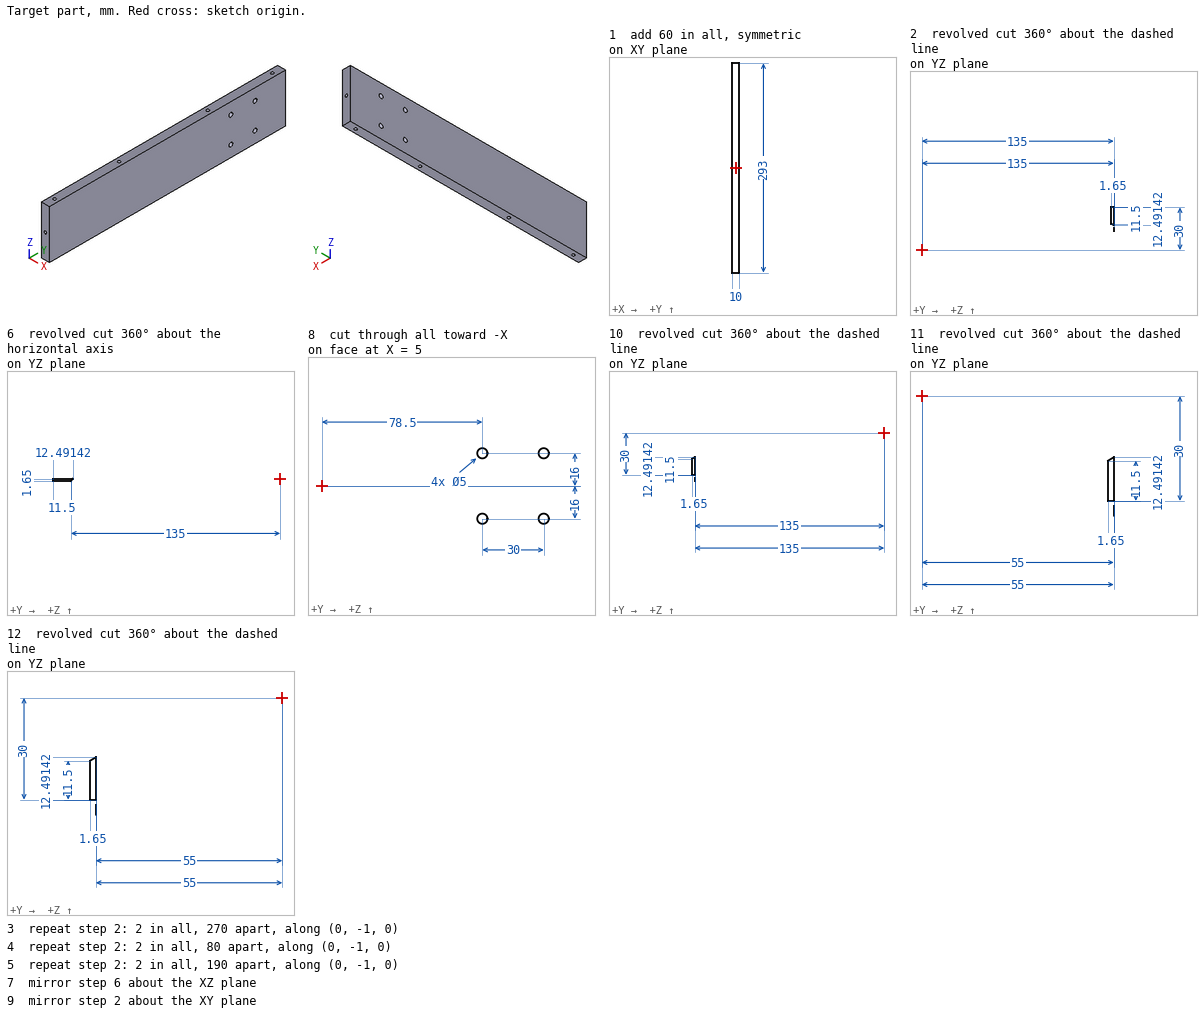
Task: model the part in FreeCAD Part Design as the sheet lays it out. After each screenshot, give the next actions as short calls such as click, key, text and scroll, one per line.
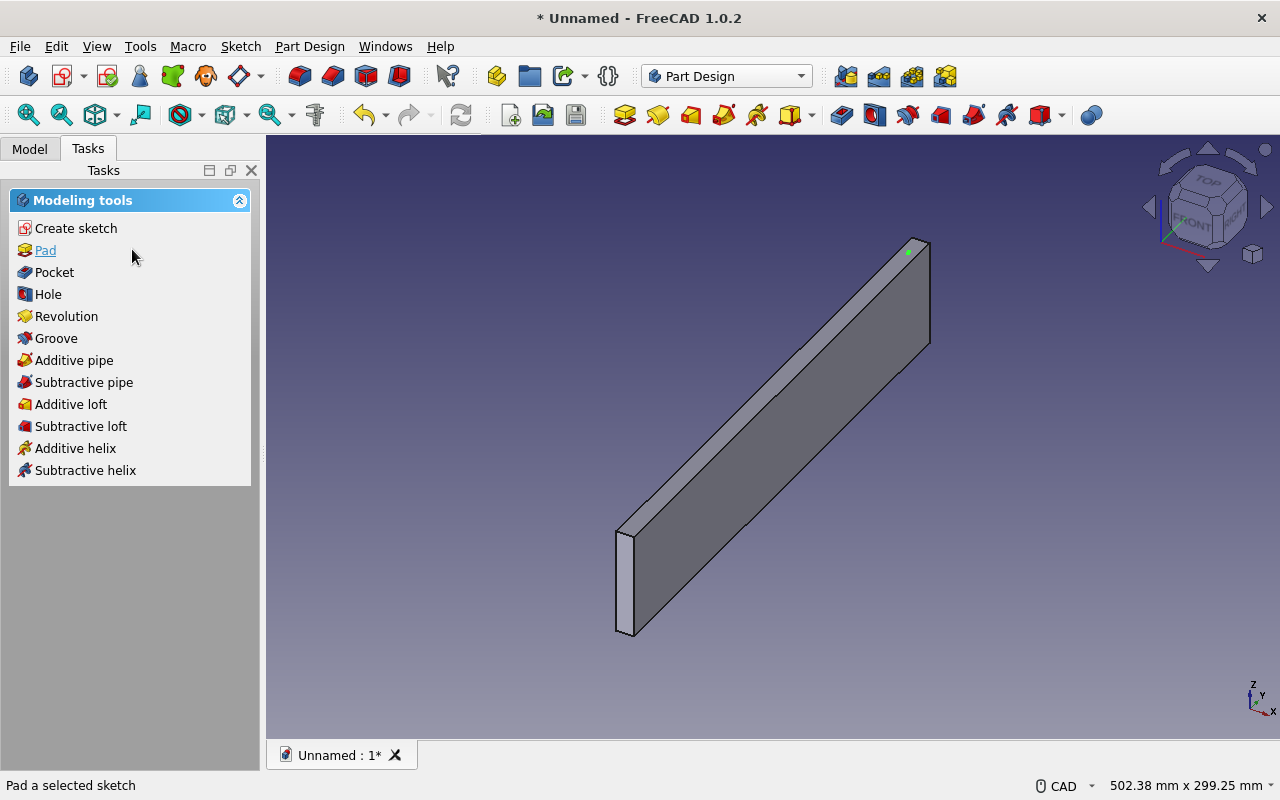
click(908, 116)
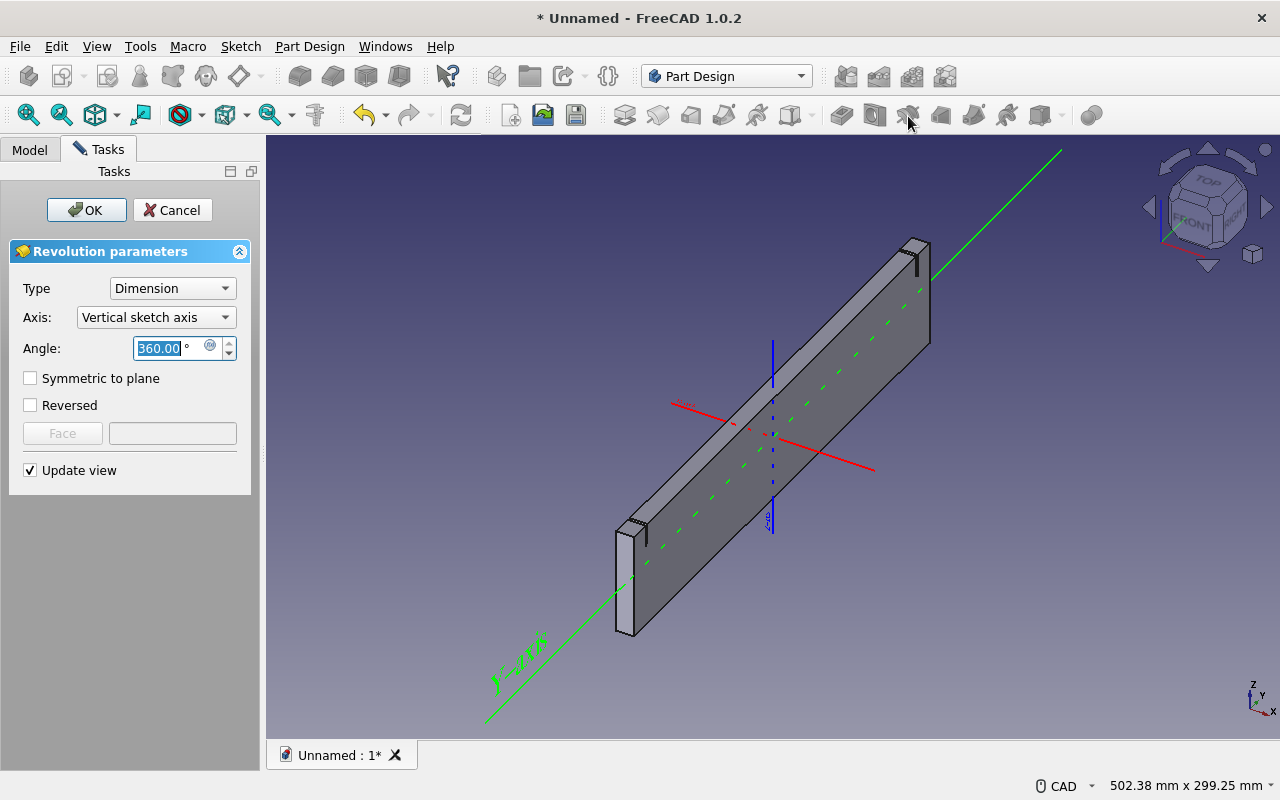
click(157, 318)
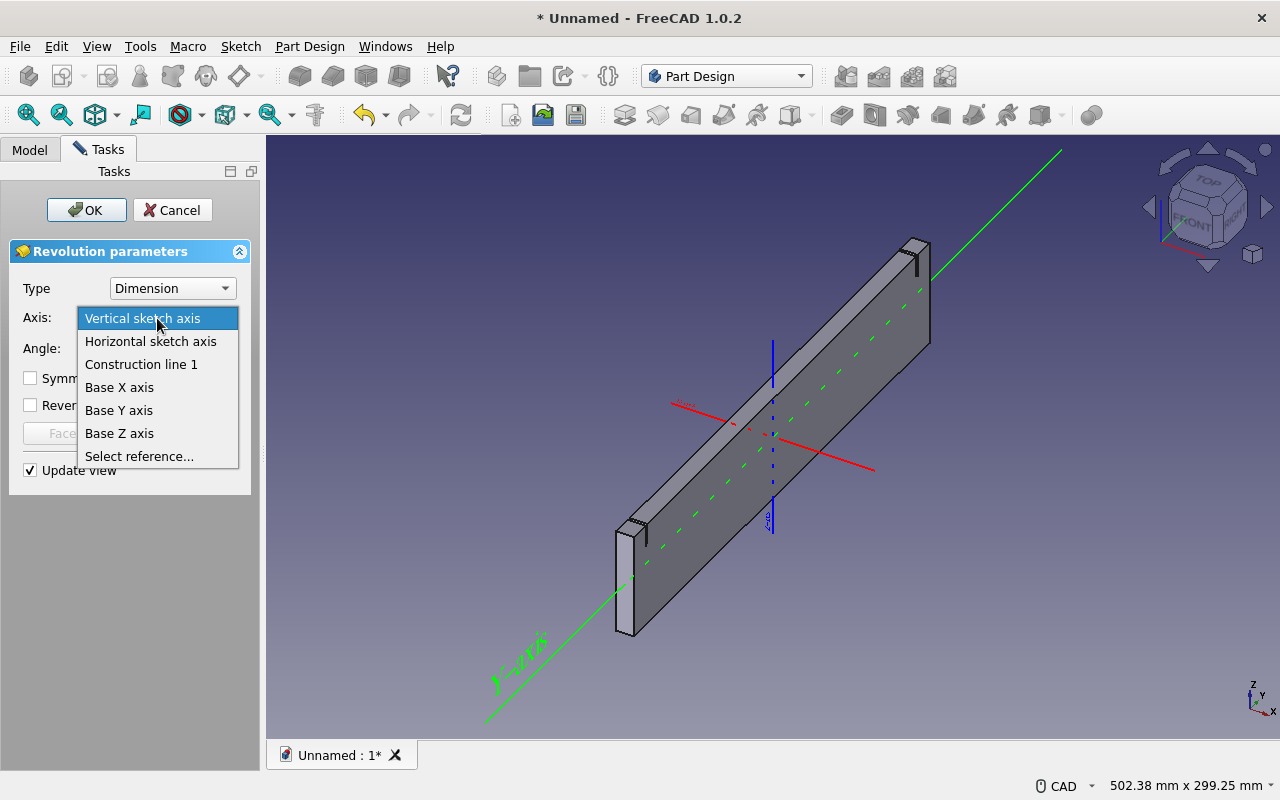
click(156, 364)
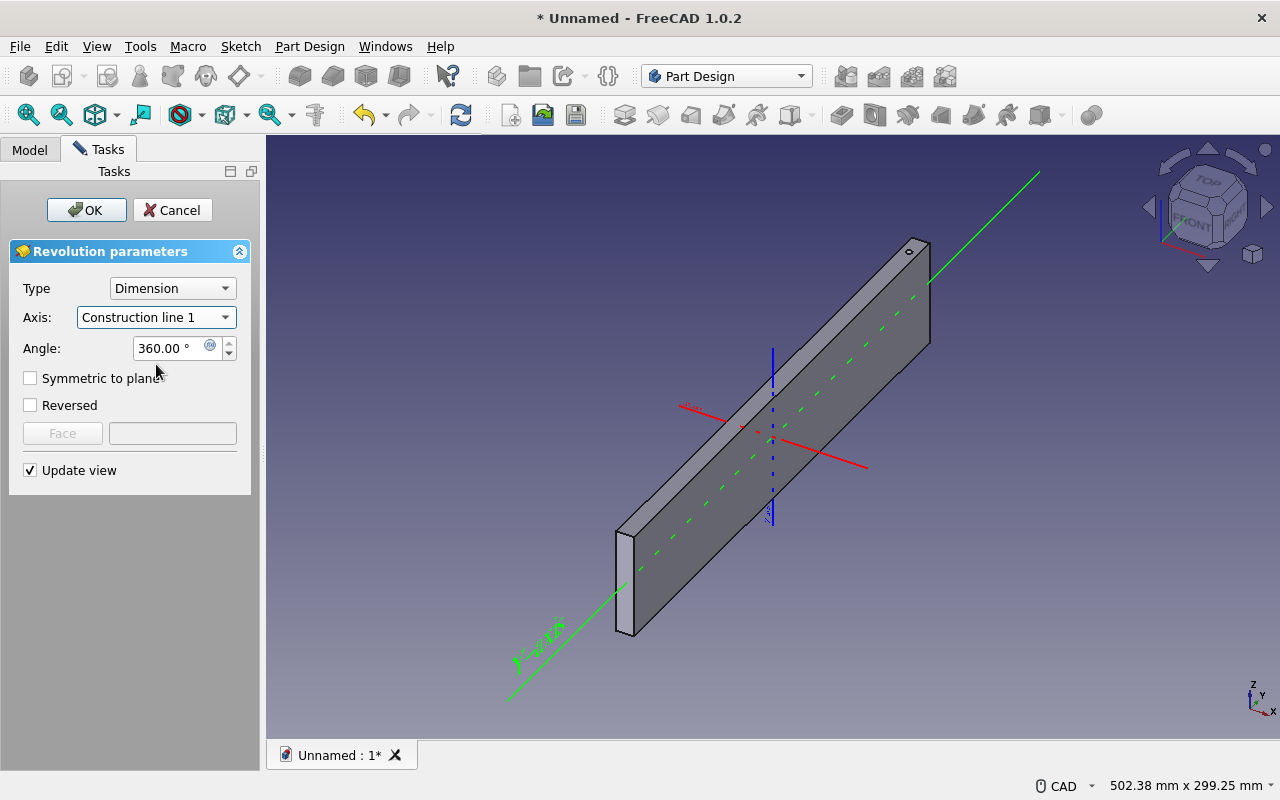
click(87, 210)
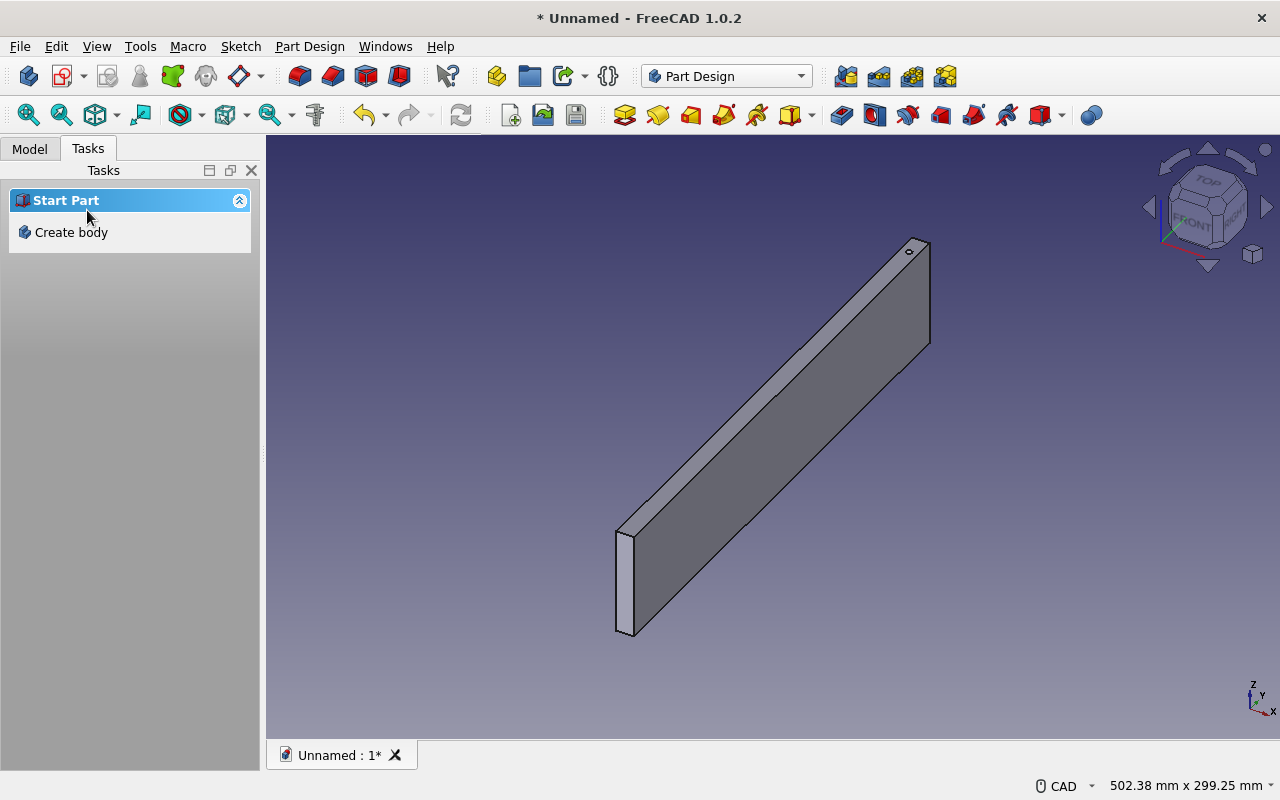
click(30, 148)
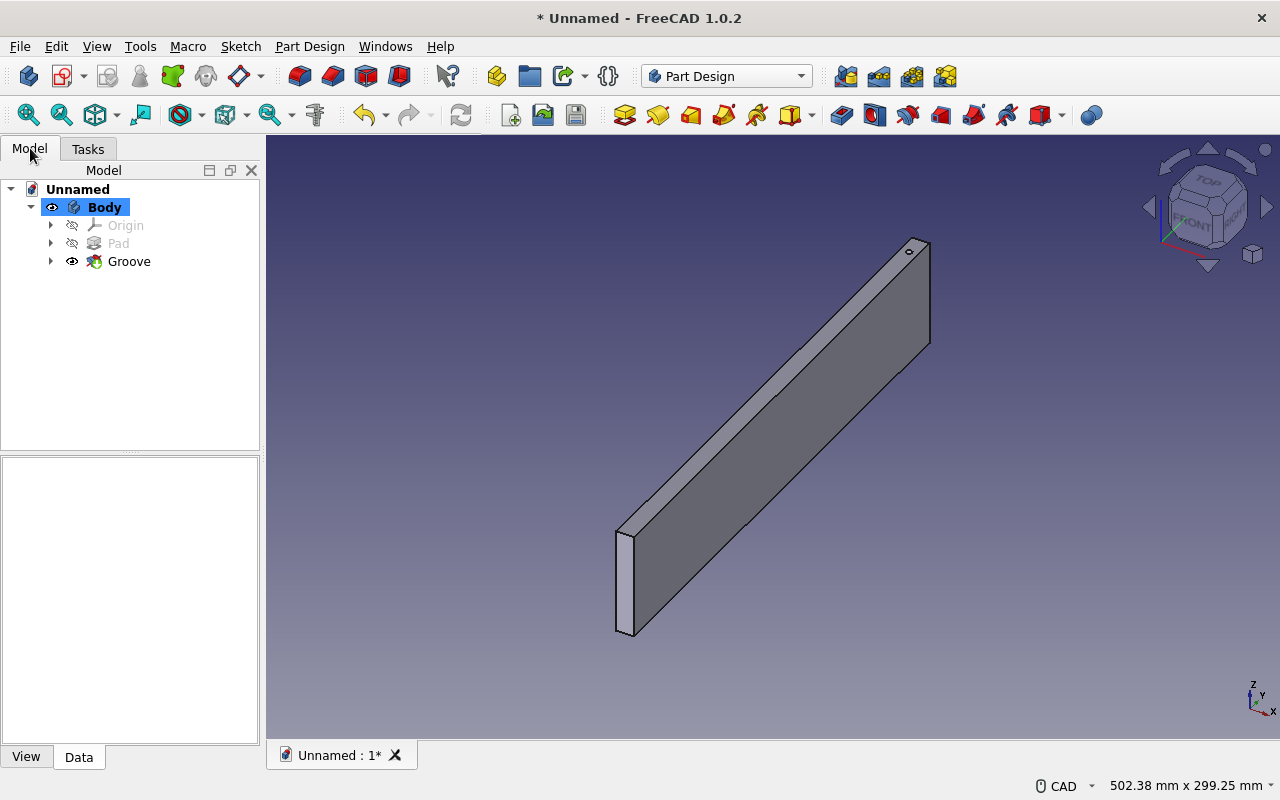
click(117, 261)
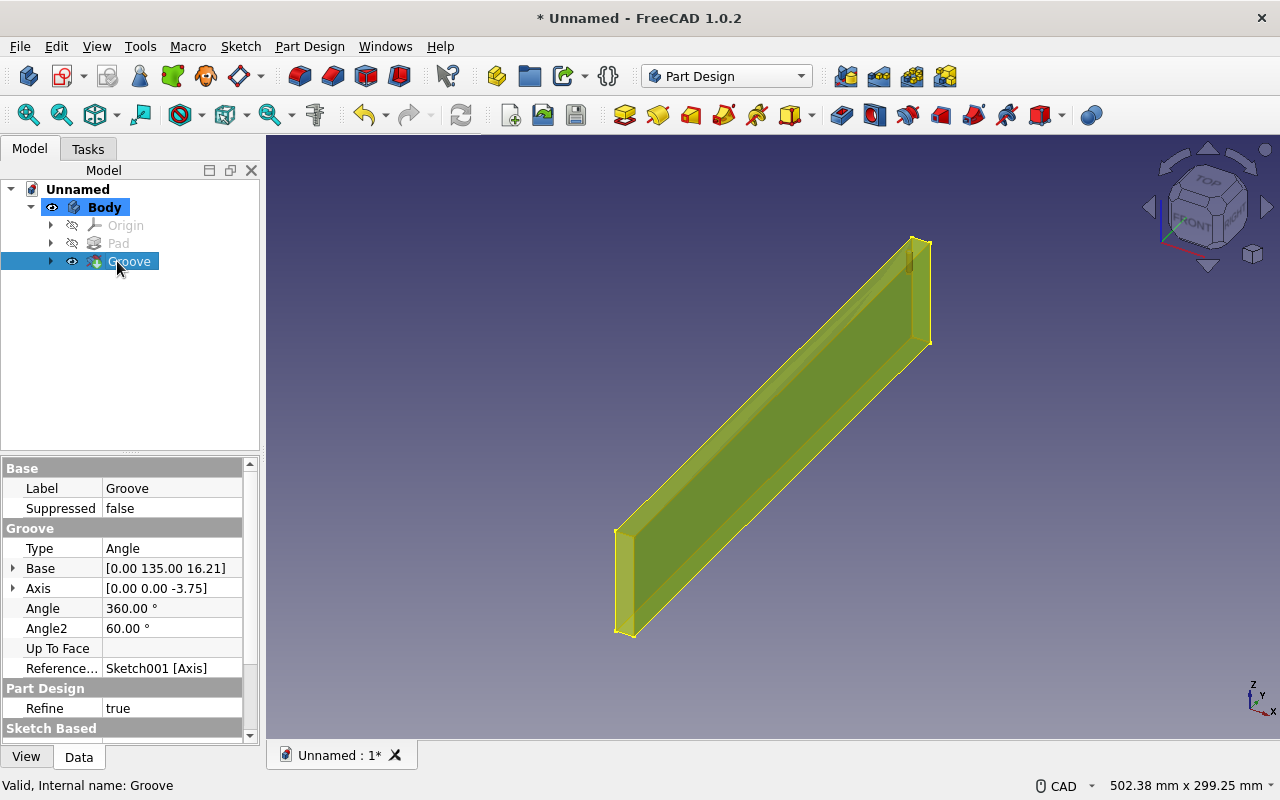
click(879, 76)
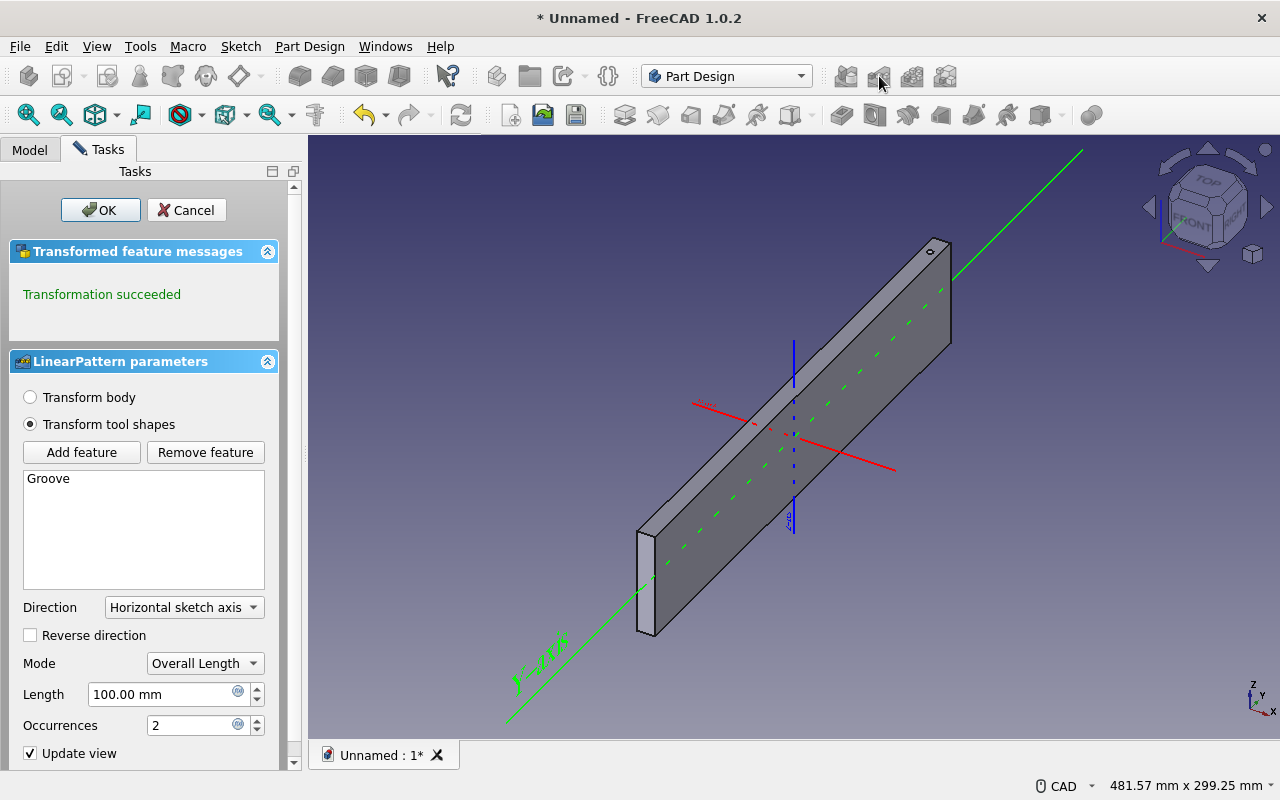
click(185, 608)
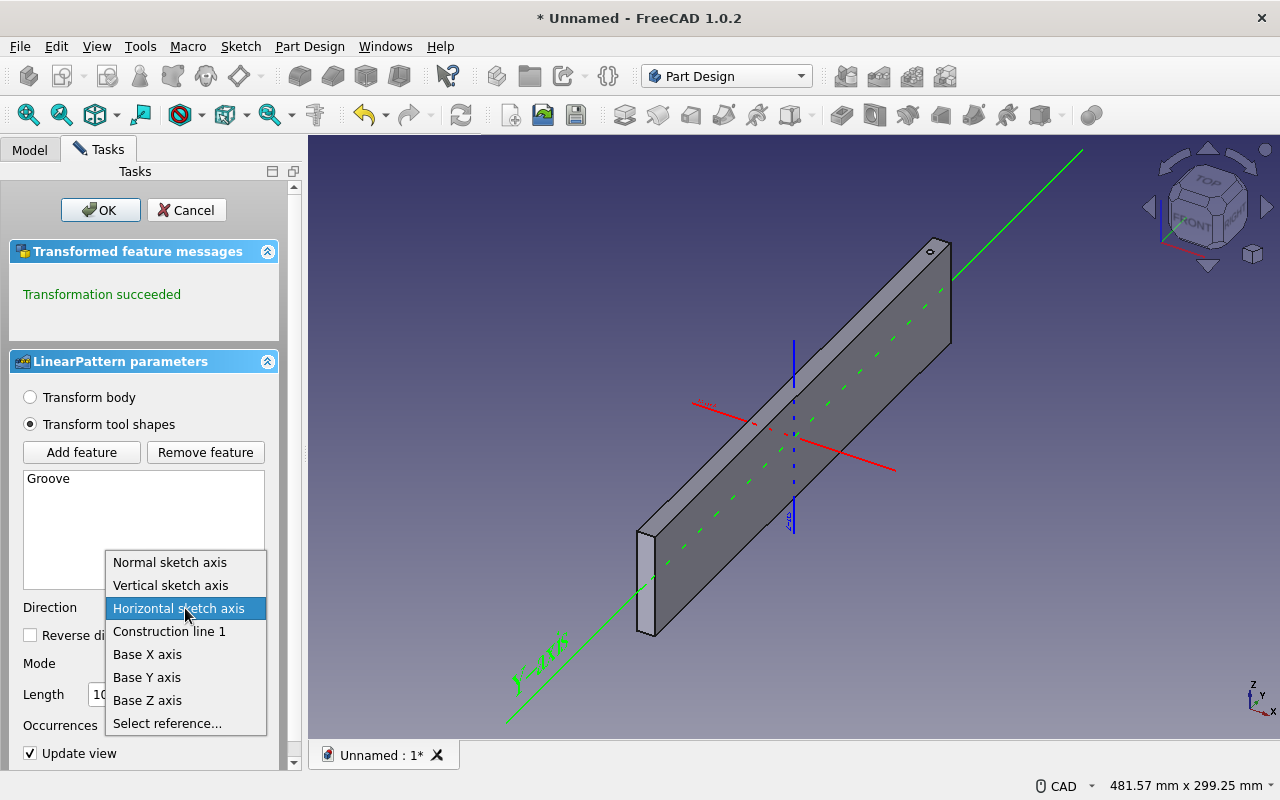
click(184, 678)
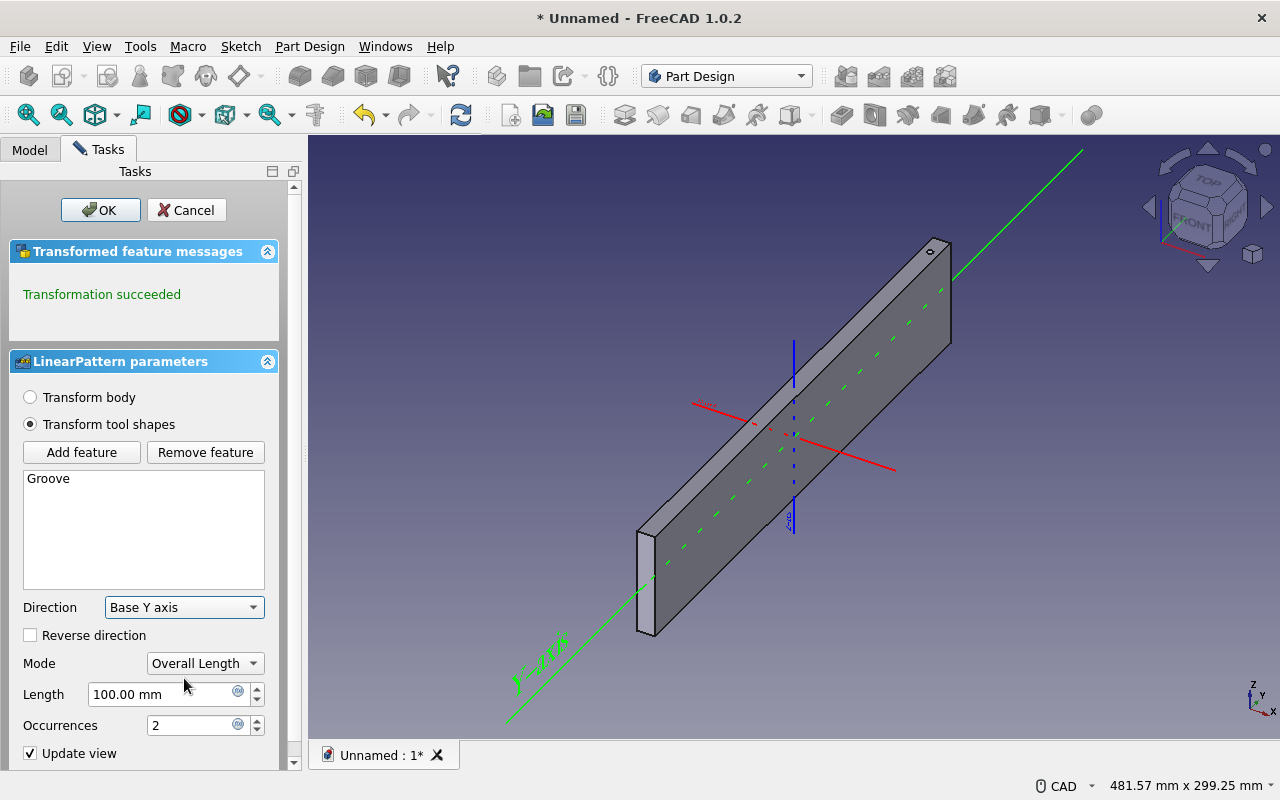
click(206, 664)